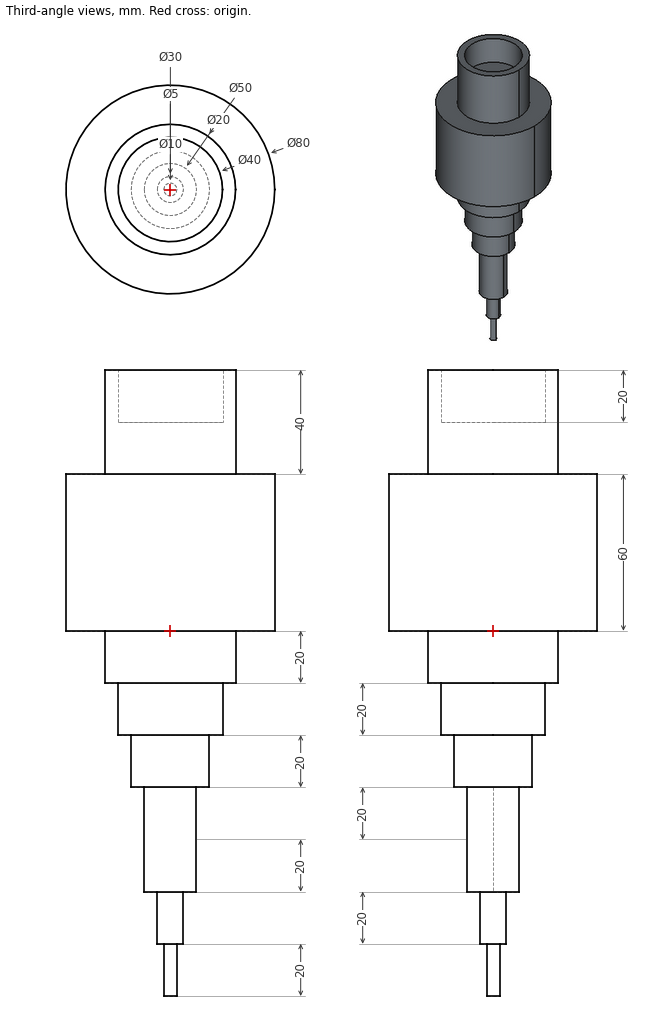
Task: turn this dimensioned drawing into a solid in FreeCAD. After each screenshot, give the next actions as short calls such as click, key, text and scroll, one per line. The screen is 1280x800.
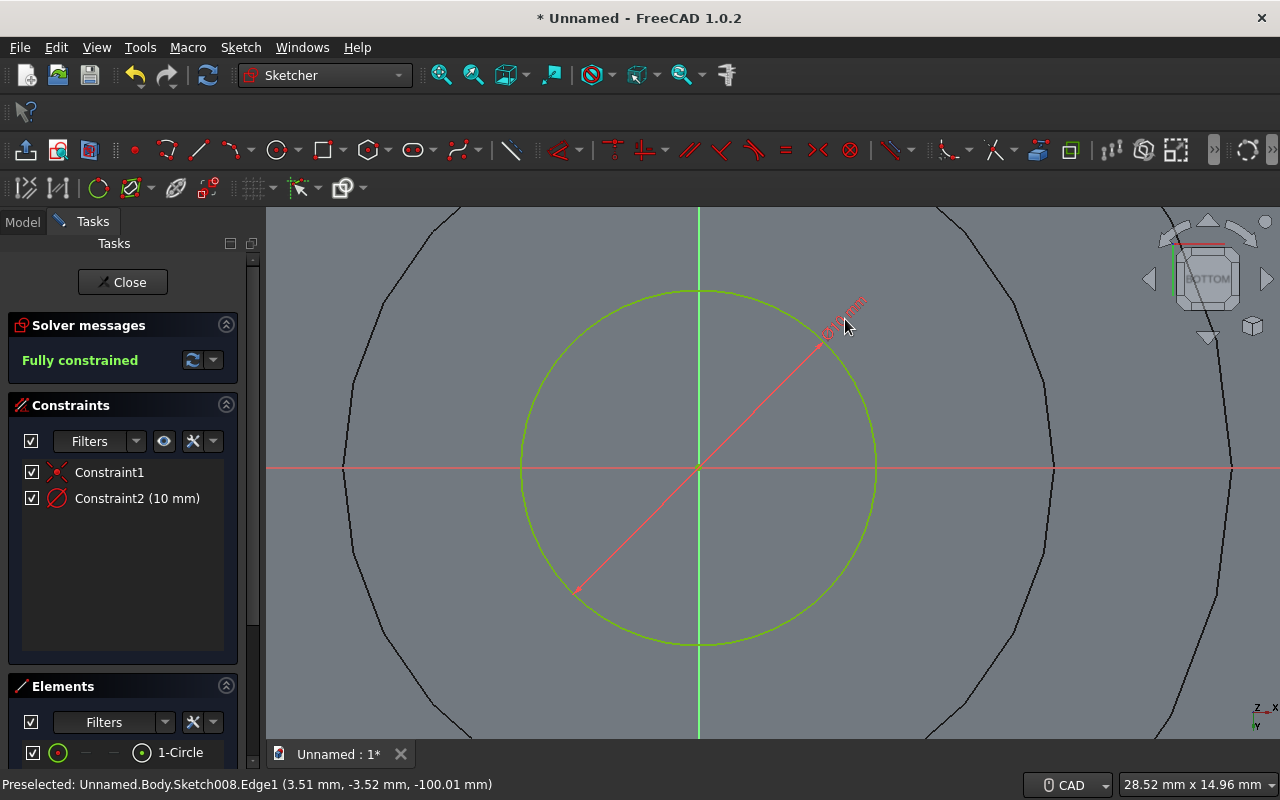
click(123, 282)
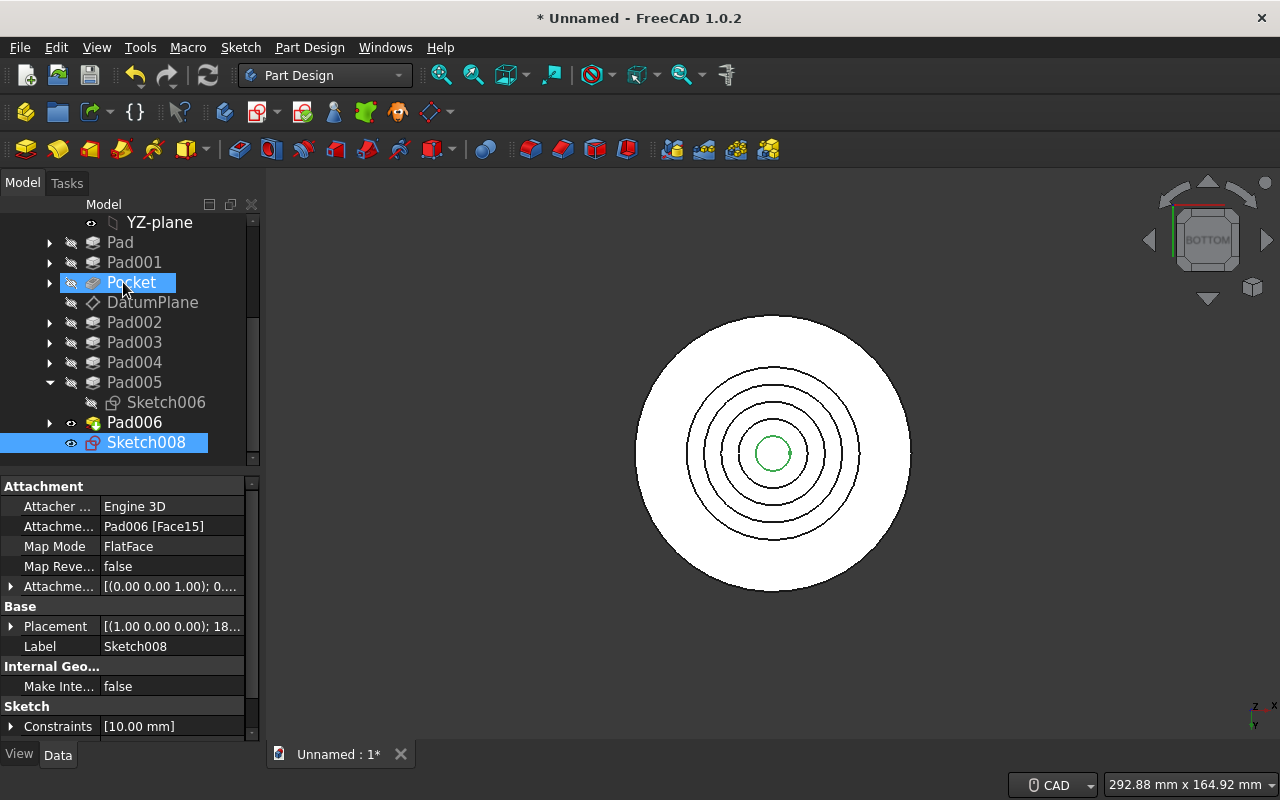
click(26, 150)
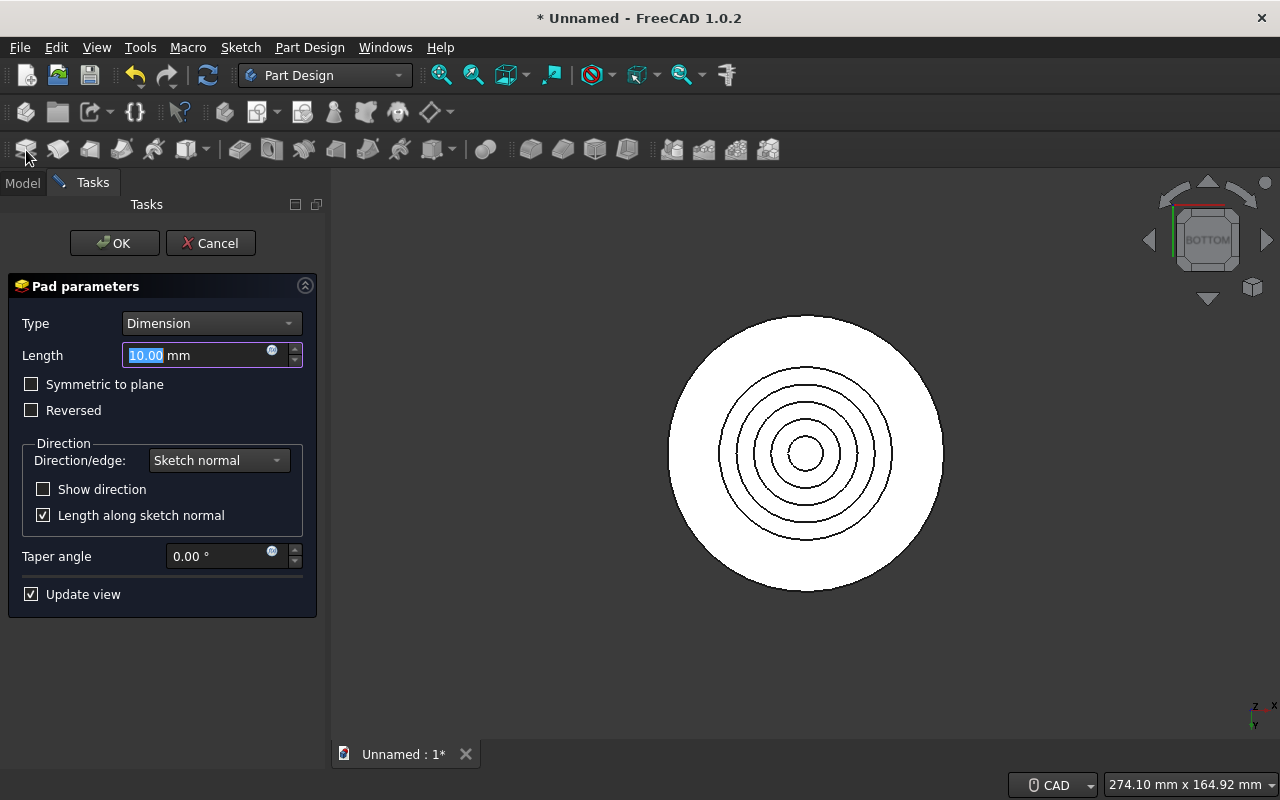
text(20)
key(Tab)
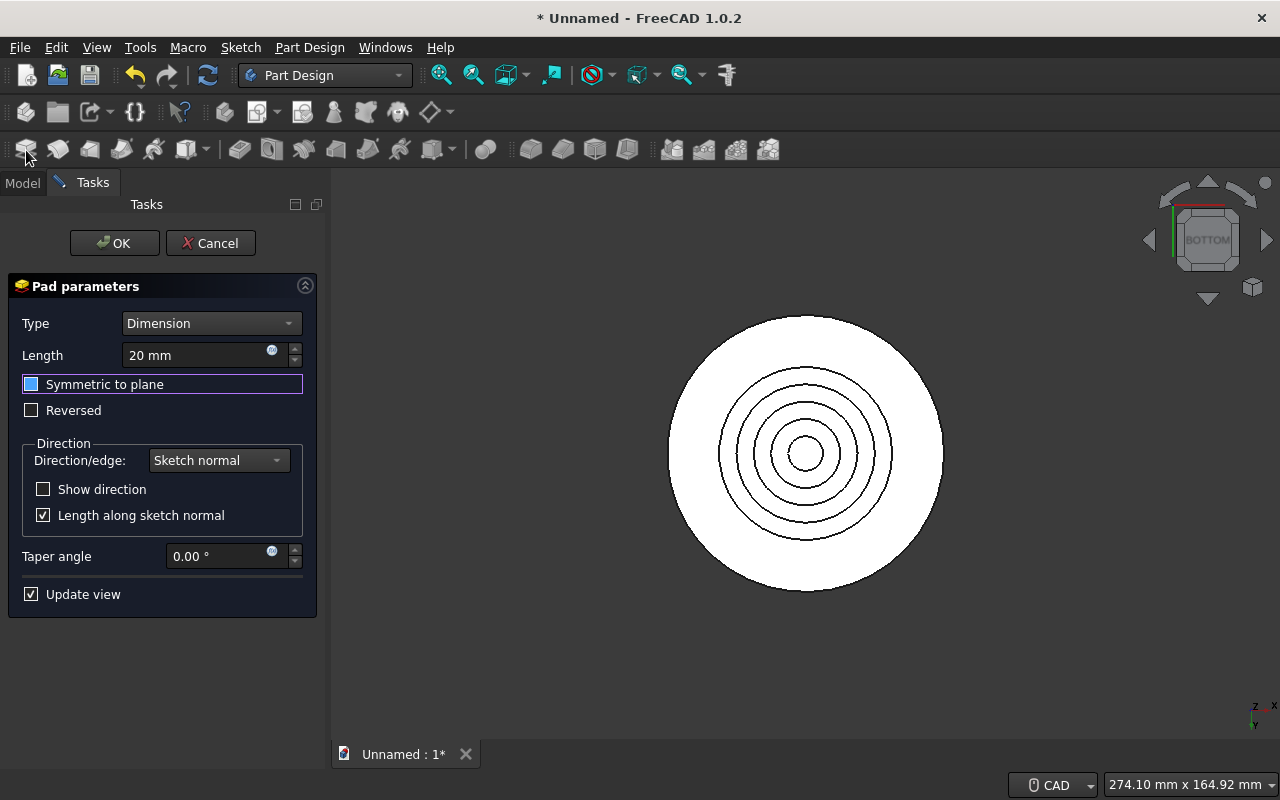
click(115, 243)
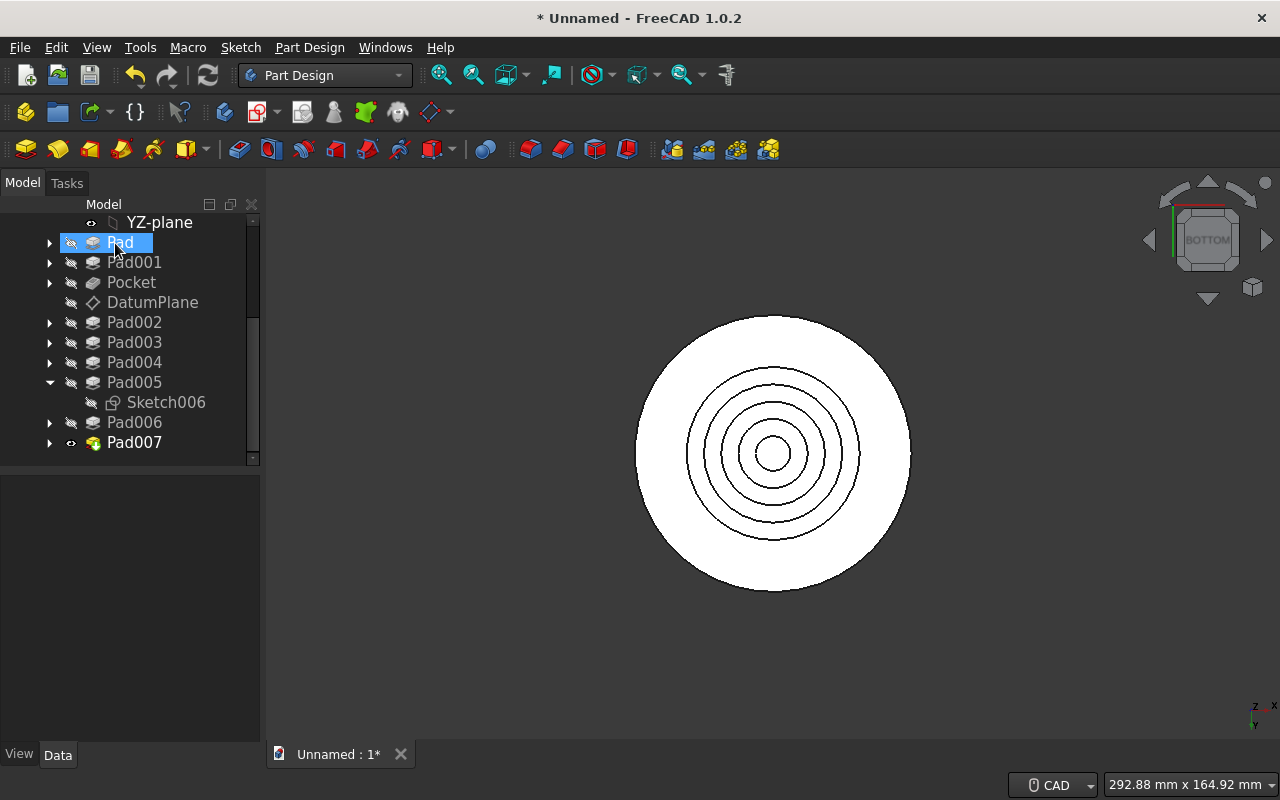
click(773, 452)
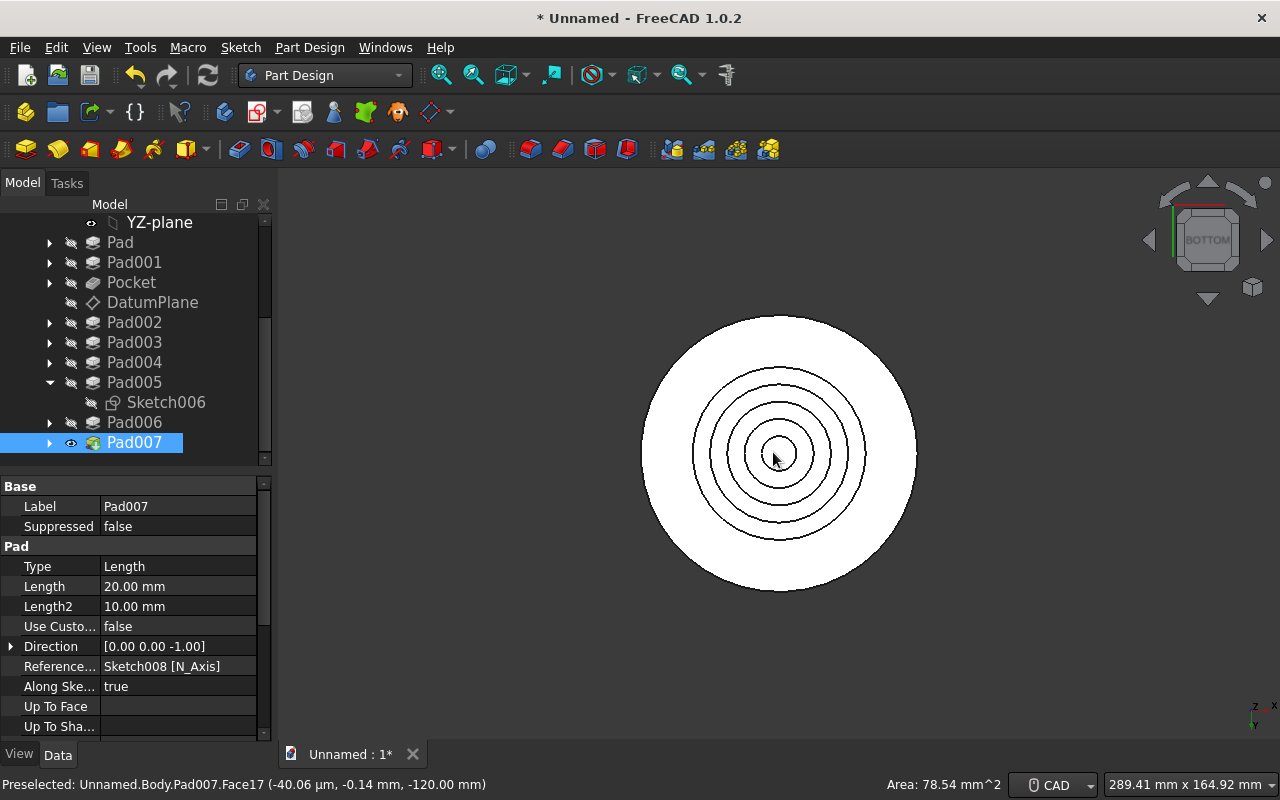
click(258, 112)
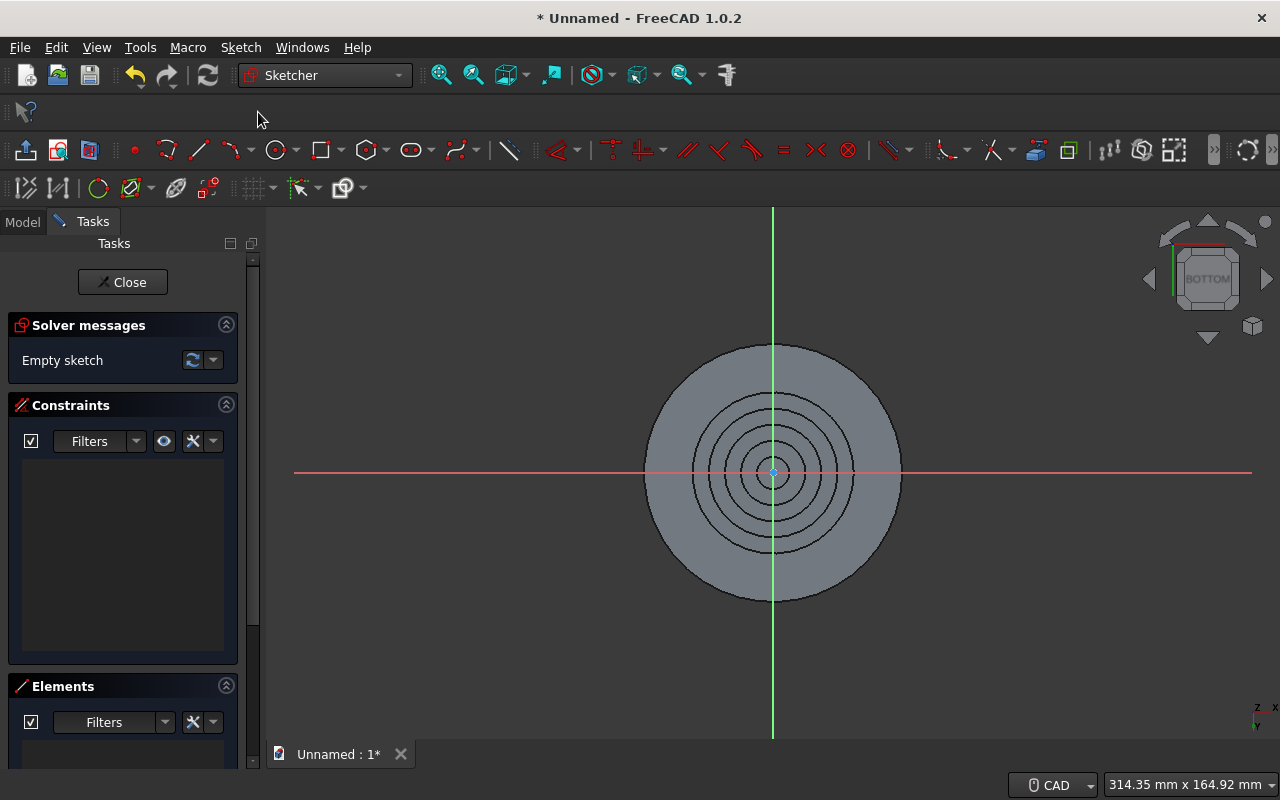
scroll(777, 473, up, 15)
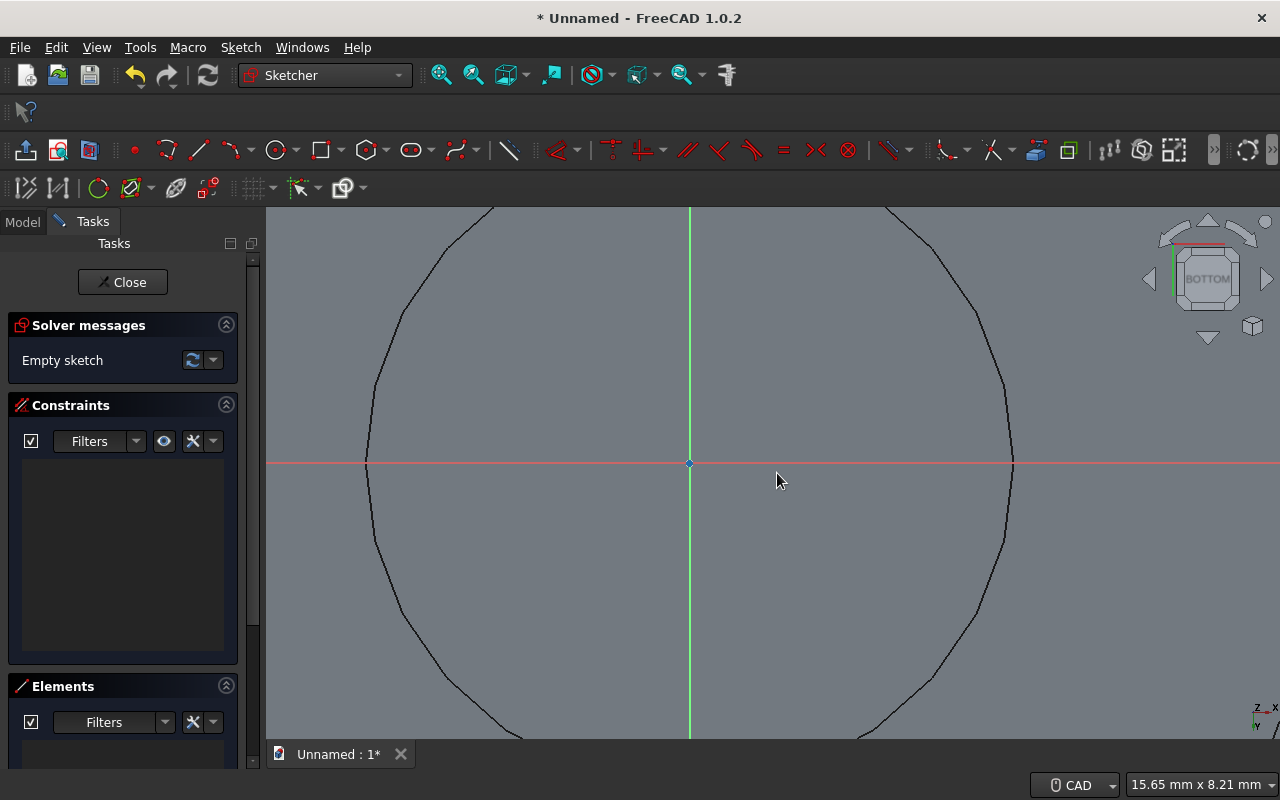
click(276, 150)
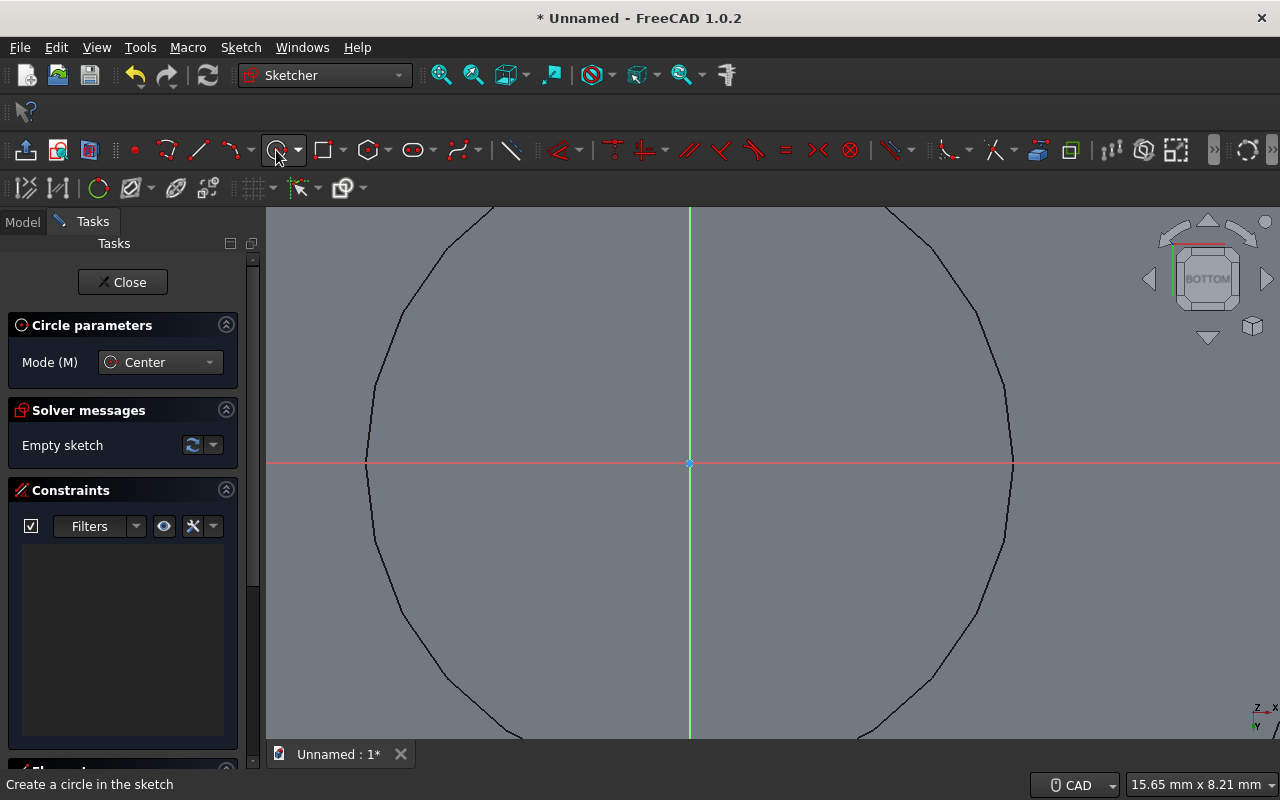
click(690, 463)
click(804, 349)
key(Escape)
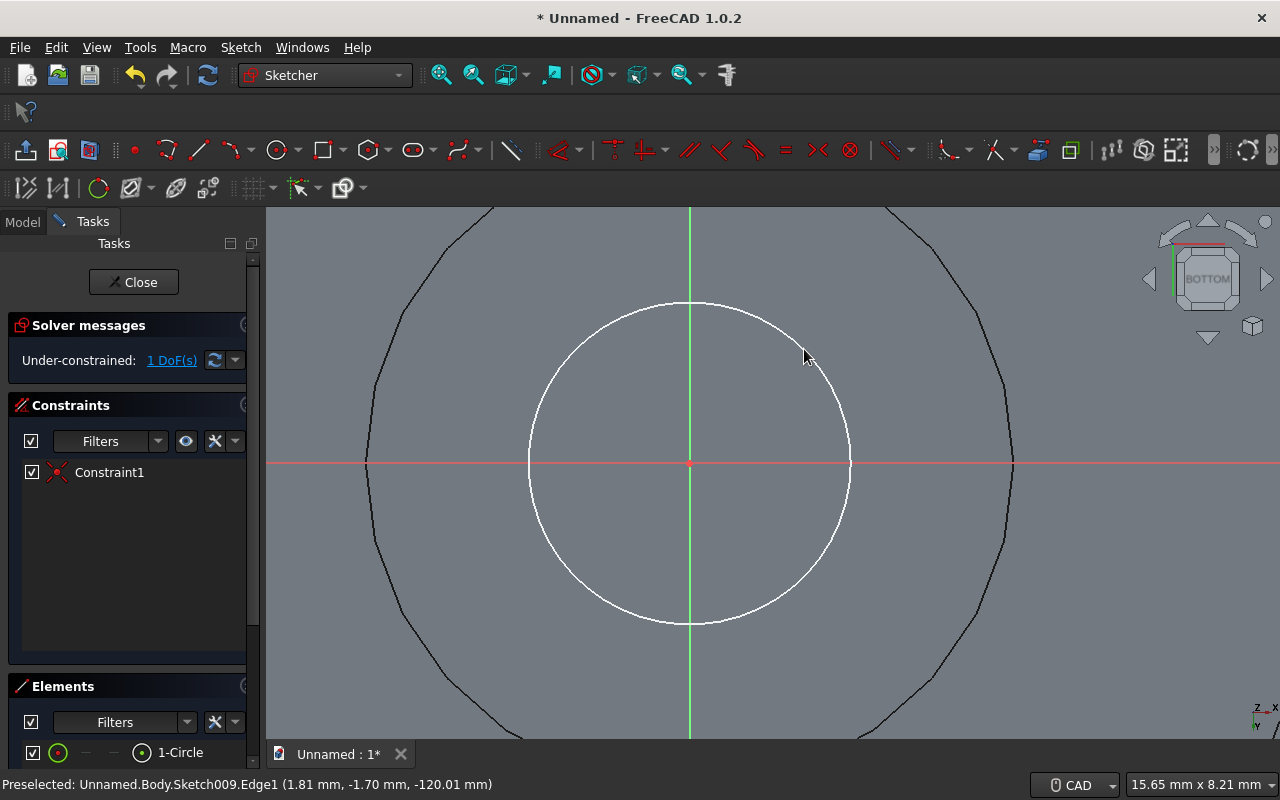
click(558, 150)